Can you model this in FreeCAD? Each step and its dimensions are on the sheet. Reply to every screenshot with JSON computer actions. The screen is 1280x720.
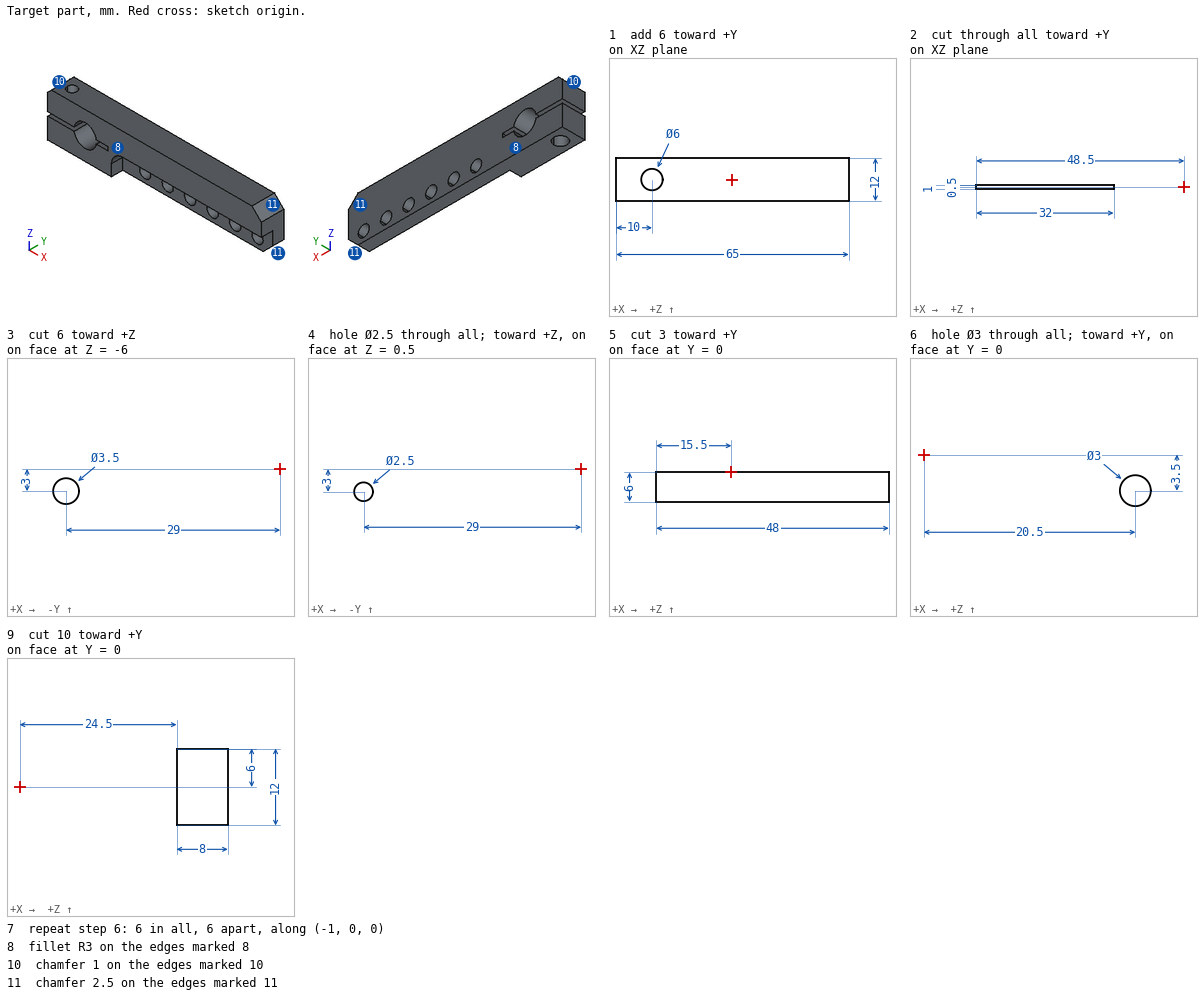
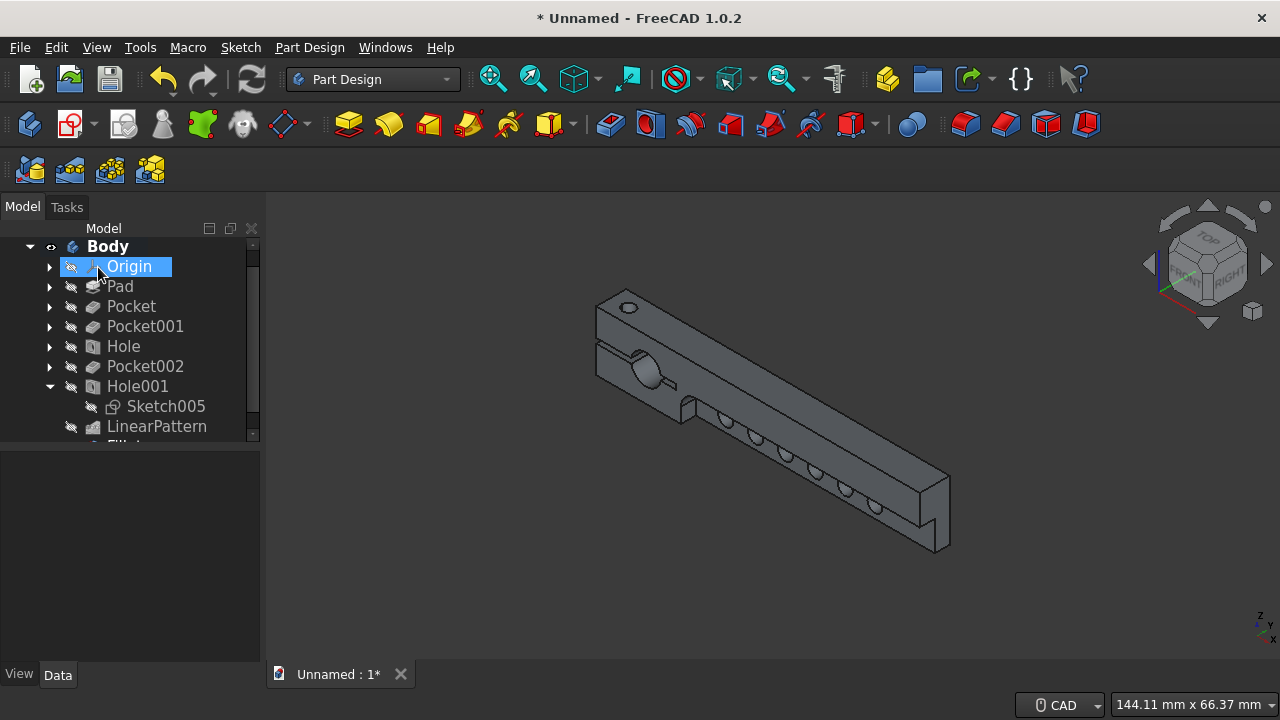
{"action": "left_click", "coordinate": [619, 373]}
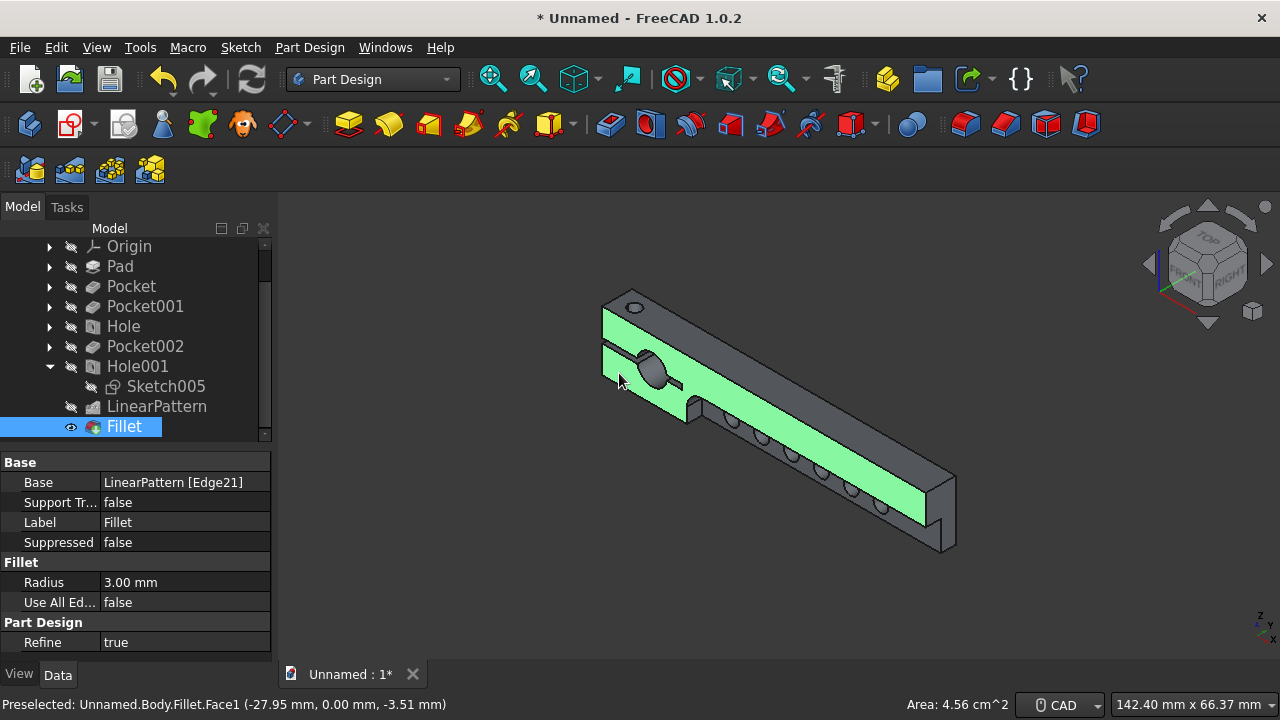
{"action": "left_click", "coordinate": [70, 124]}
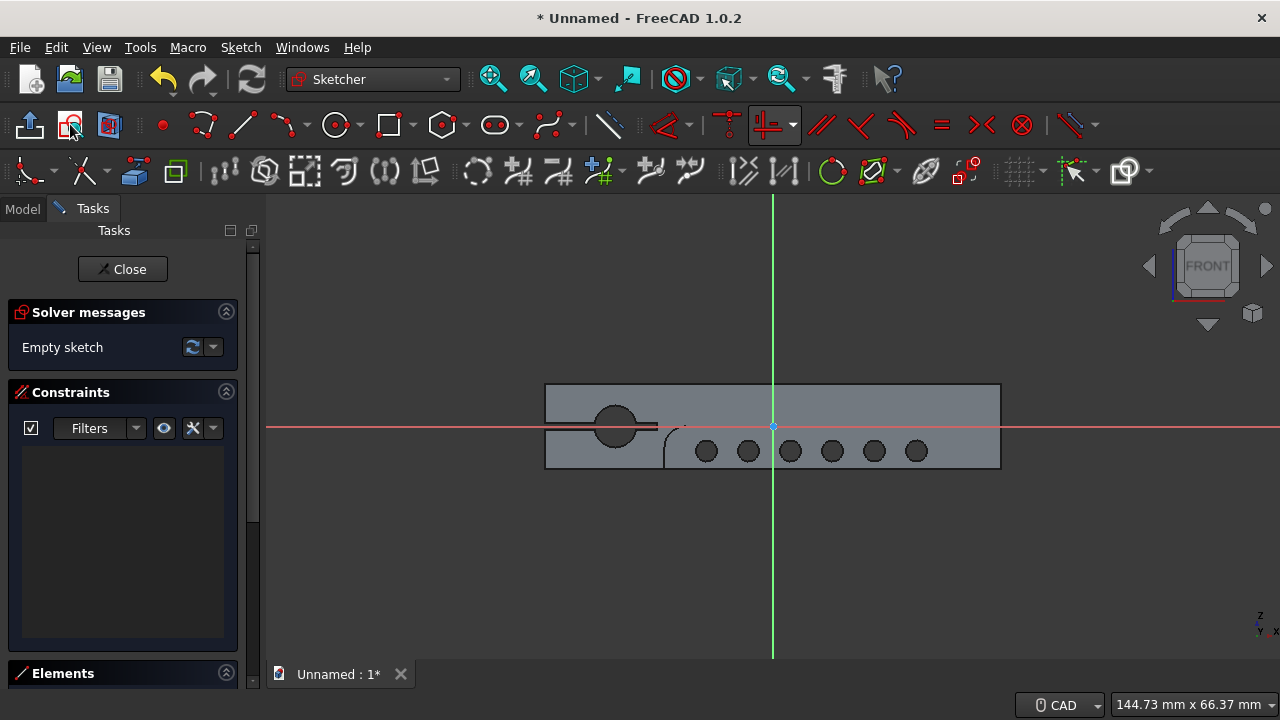
{"action": "scroll", "coordinate": [1088, 426], "scroll_direction": "up", "scroll_amount": 6}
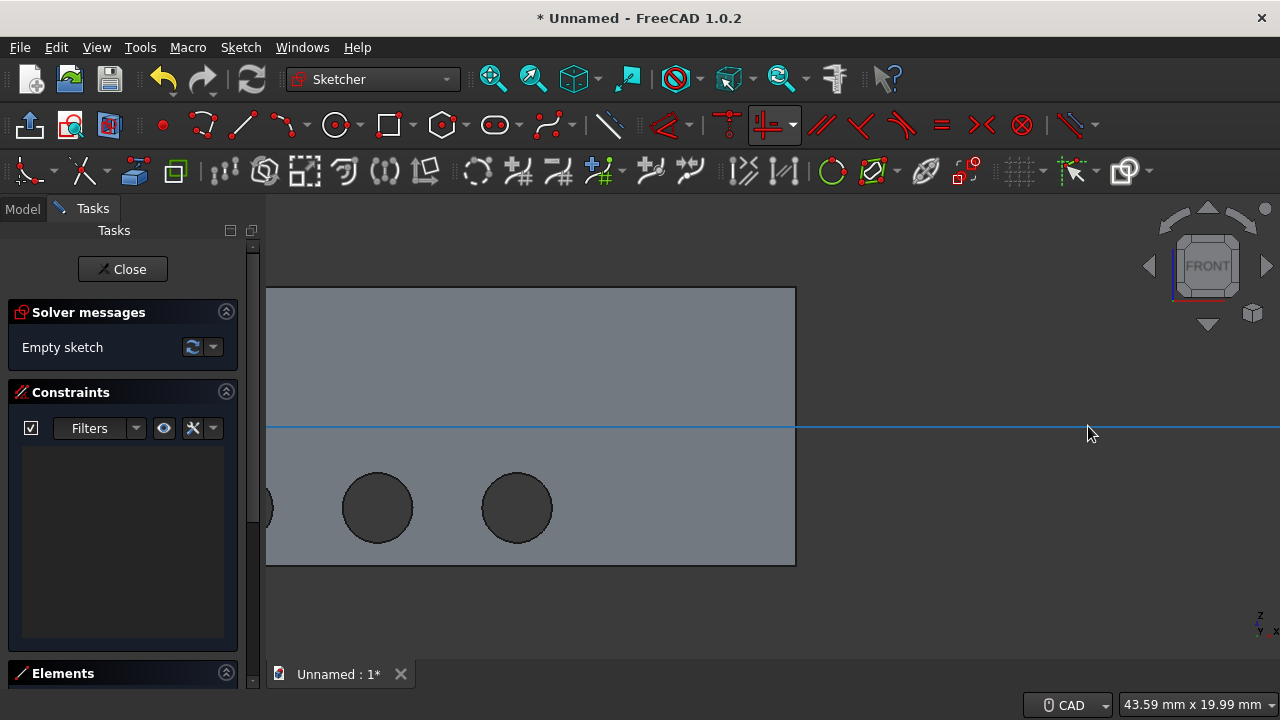
{"action": "left_click", "coordinate": [390, 126]}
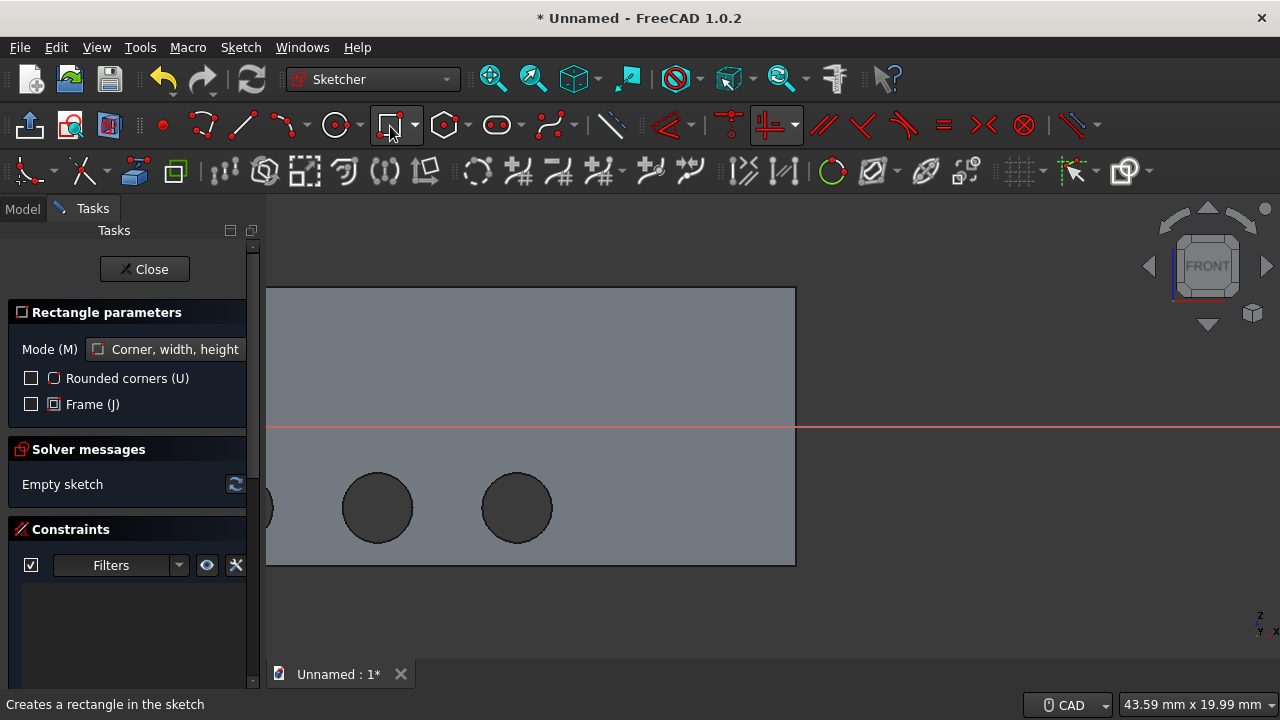
{"action": "left_click", "coordinate": [610, 287]}
{"action": "left_click", "coordinate": [796, 566]}
{"action": "key", "text": "Escape"}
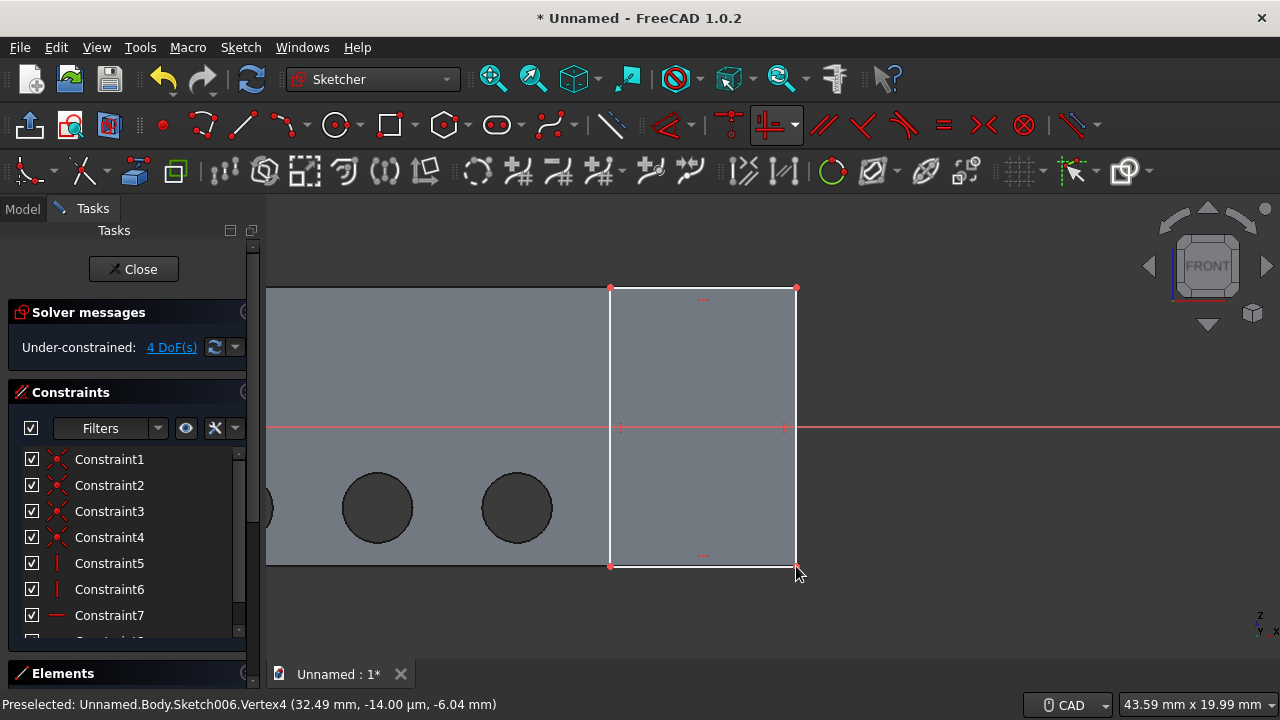
{"action": "key", "text": "d"}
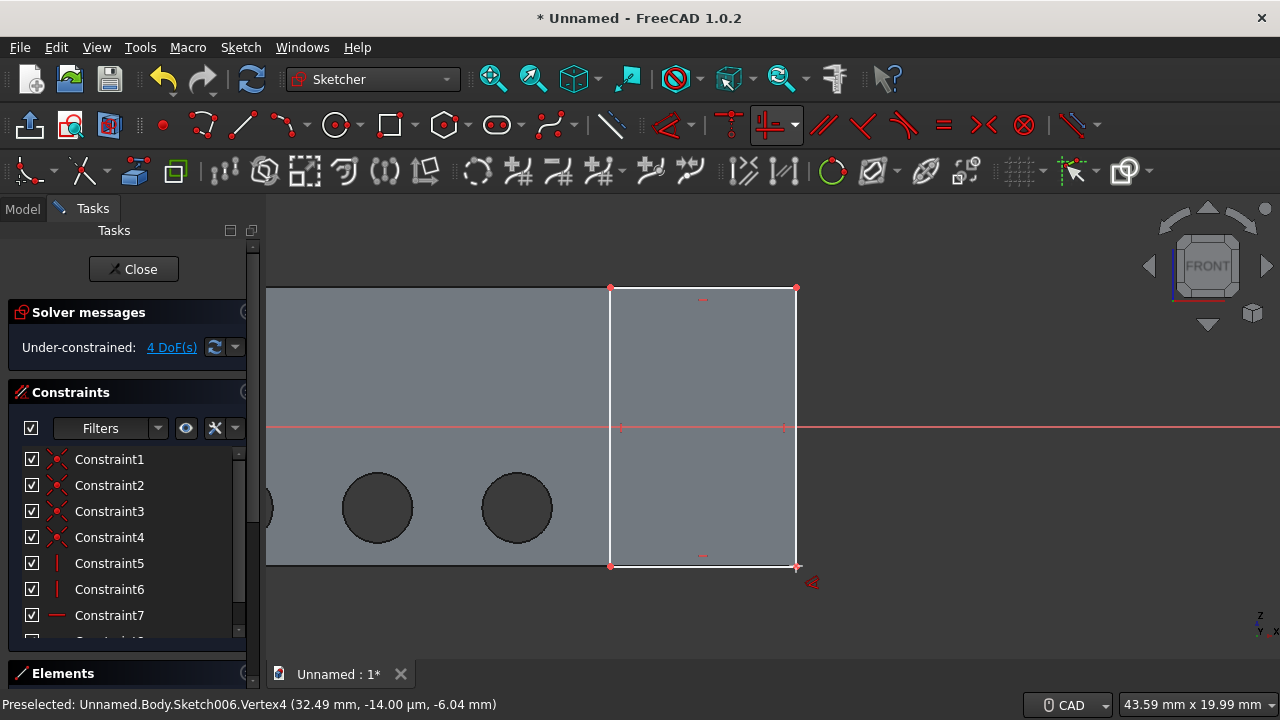
{"action": "left_click", "coordinate": [666, 567]}
{"action": "left_click", "coordinate": [703, 601]}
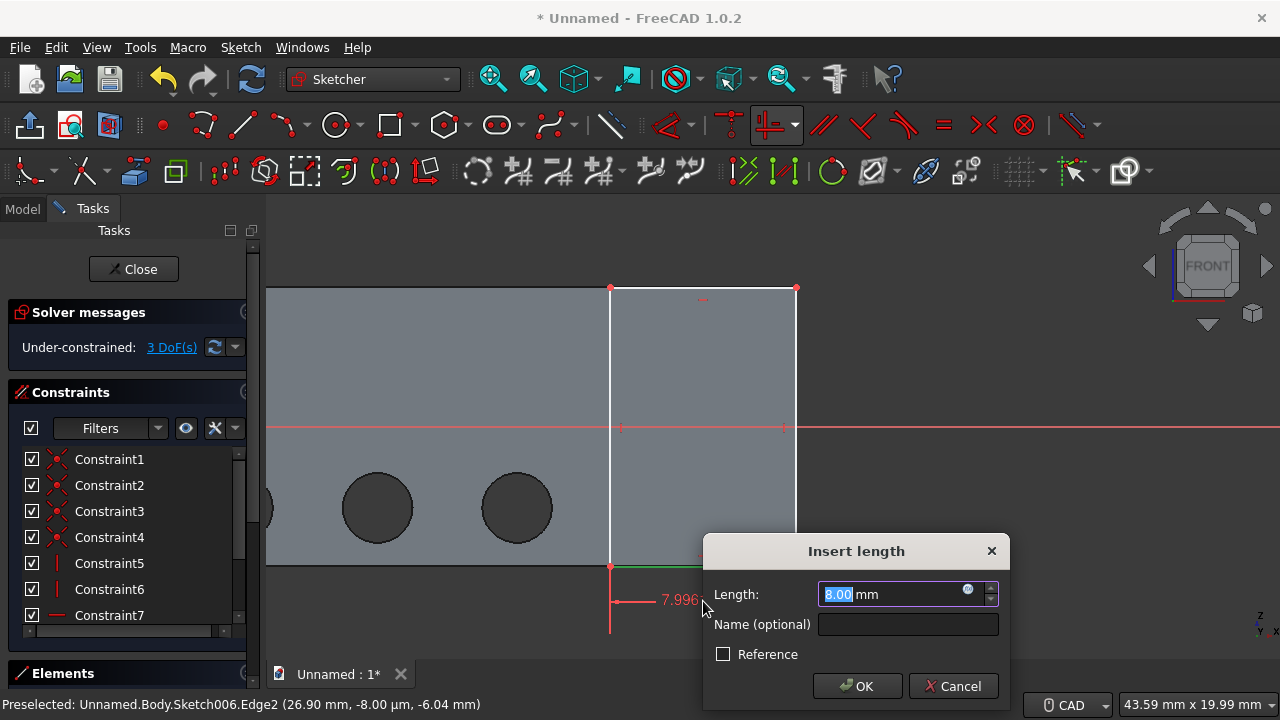
{"action": "type", "text": "8"}
{"action": "key", "text": "Return"}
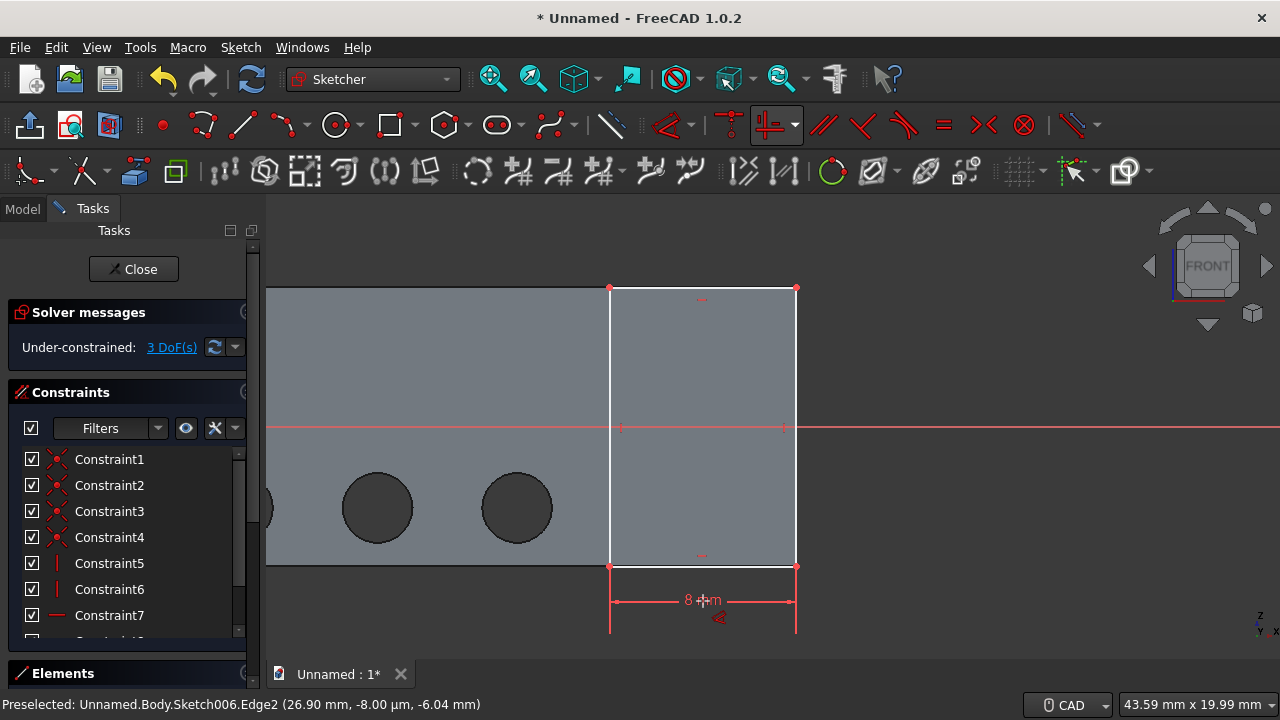
{"action": "left_click", "coordinate": [610, 372]}
{"action": "left_click", "coordinate": [576, 363]}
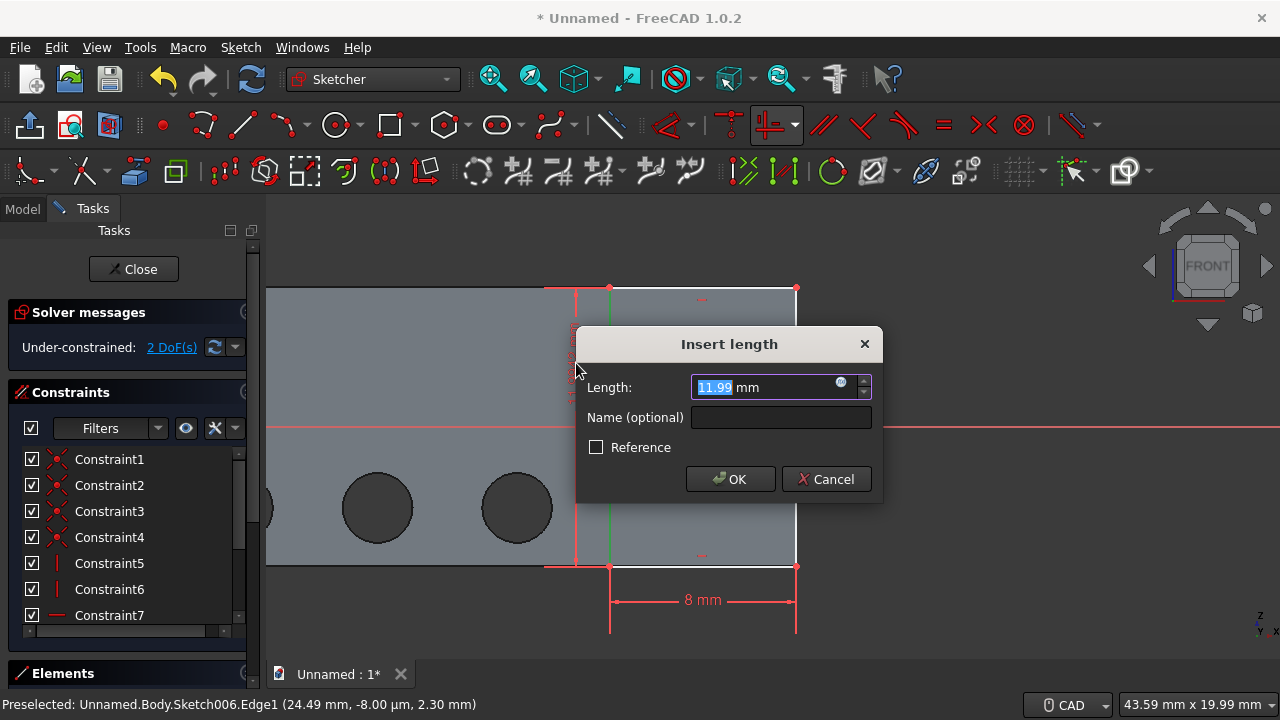
{"action": "type", "text": "12"}
{"action": "key", "text": "Return"}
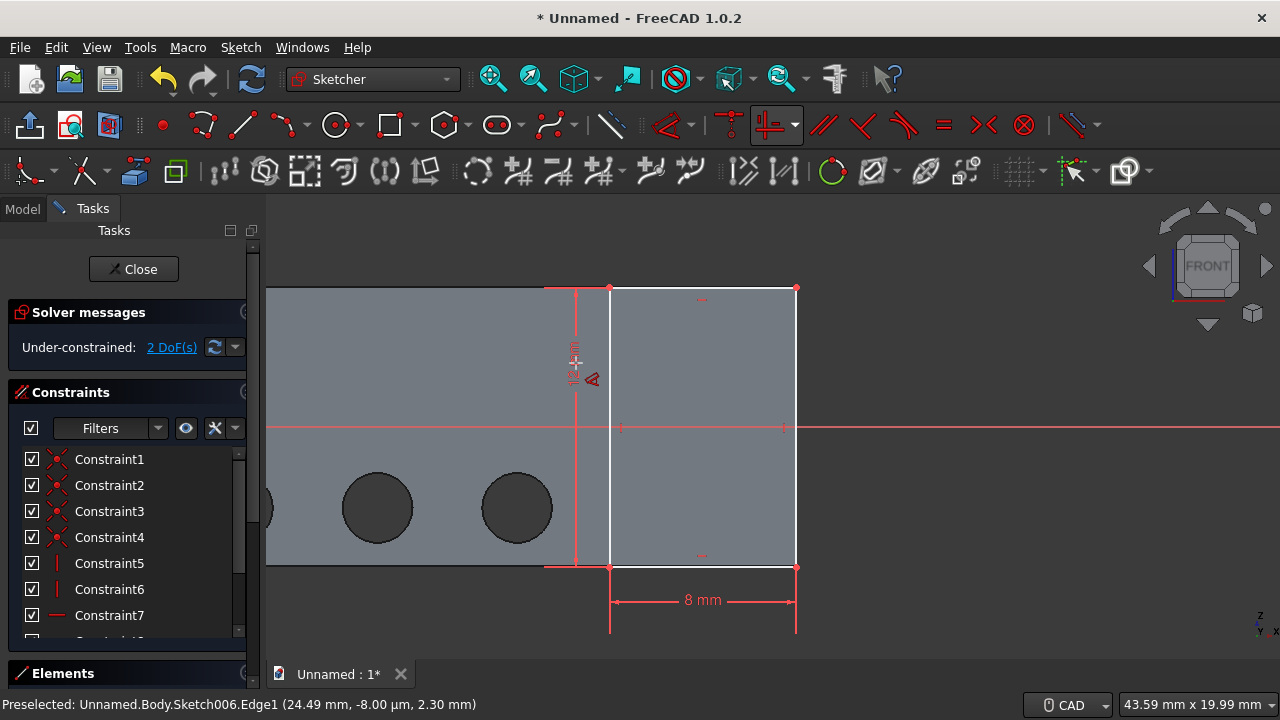
{"action": "left_click", "coordinate": [610, 288]}
{"action": "left_click", "coordinate": [644, 325]}